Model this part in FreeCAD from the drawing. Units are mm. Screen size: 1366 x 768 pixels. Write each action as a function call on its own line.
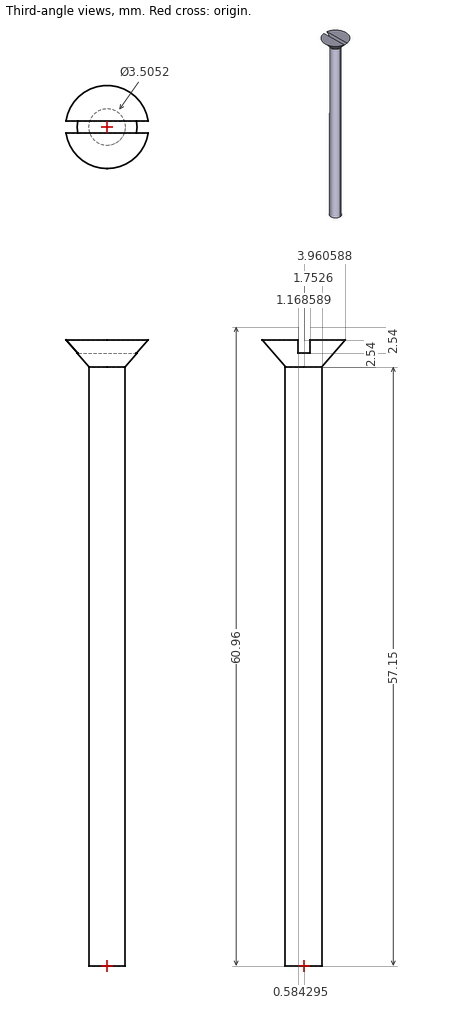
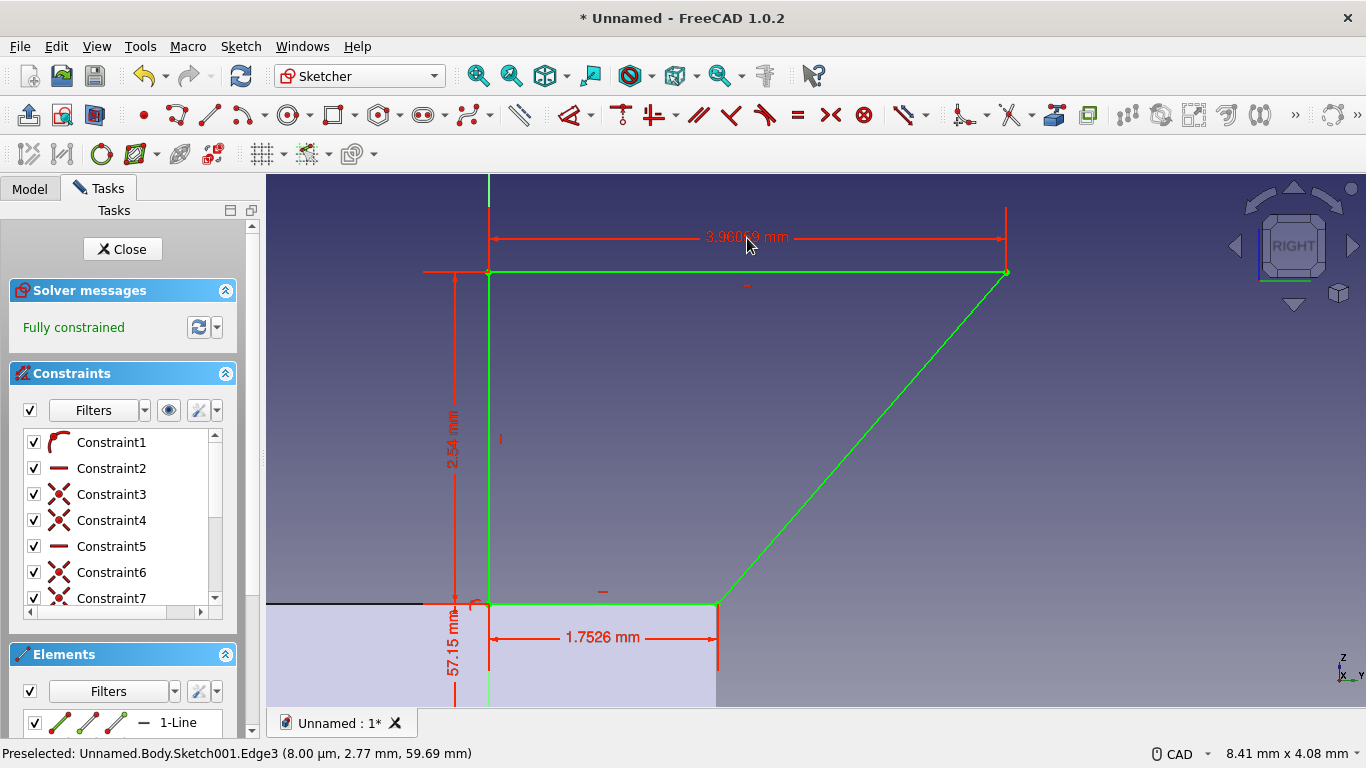
click(123, 249)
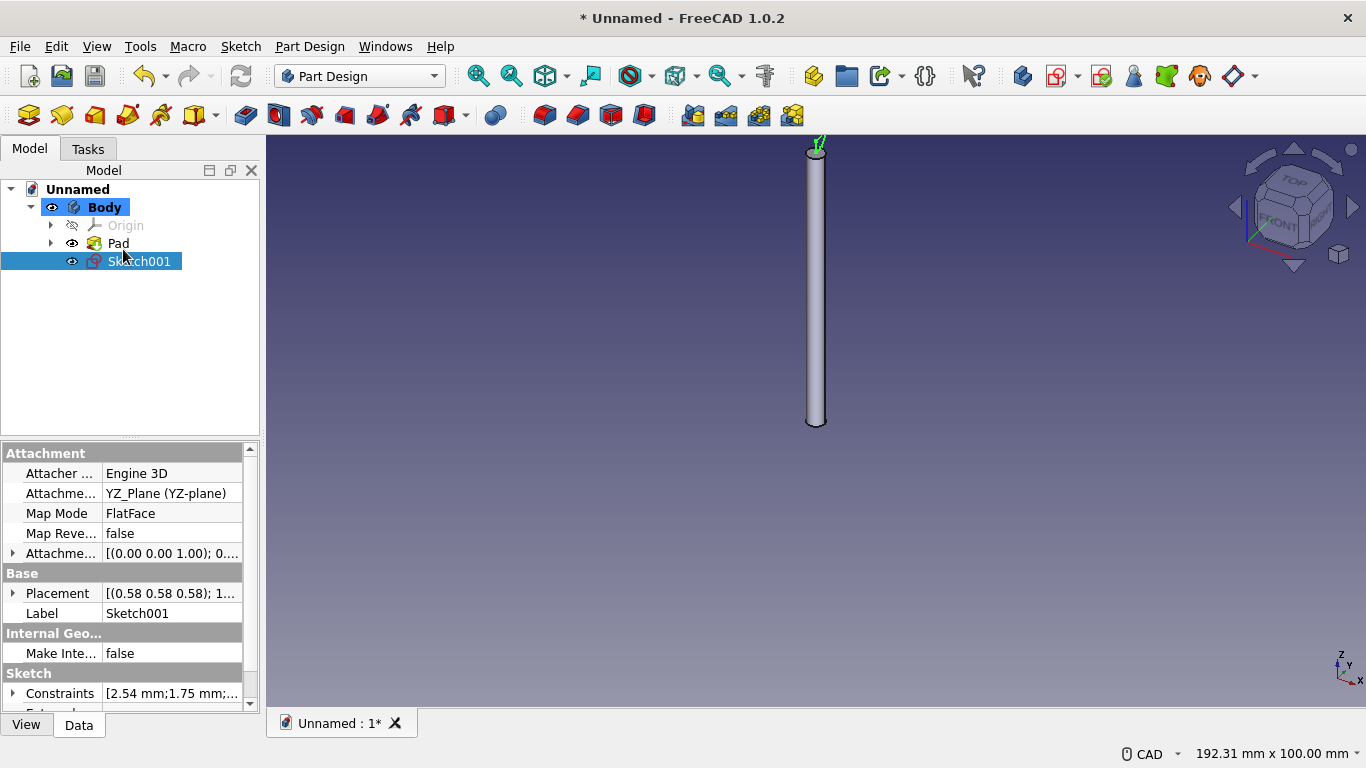
click(62, 116)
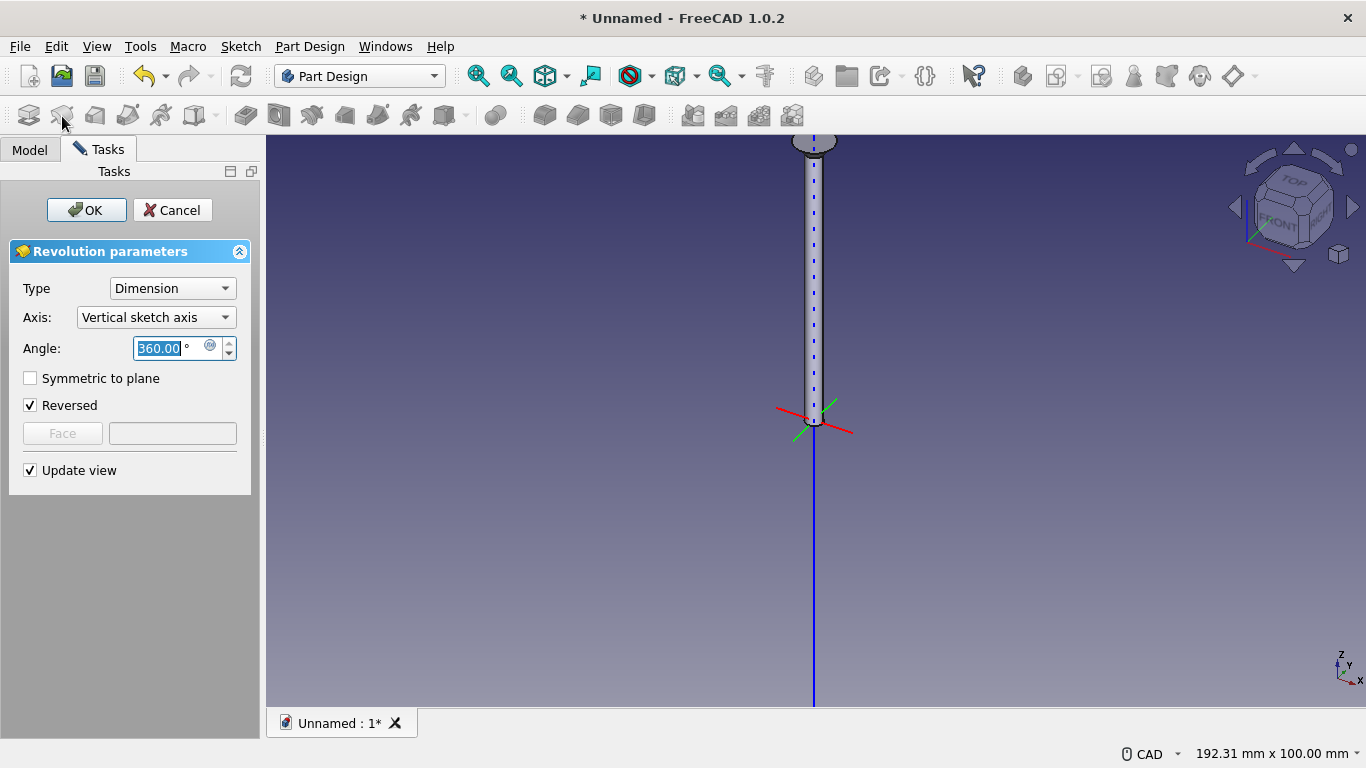
click(87, 210)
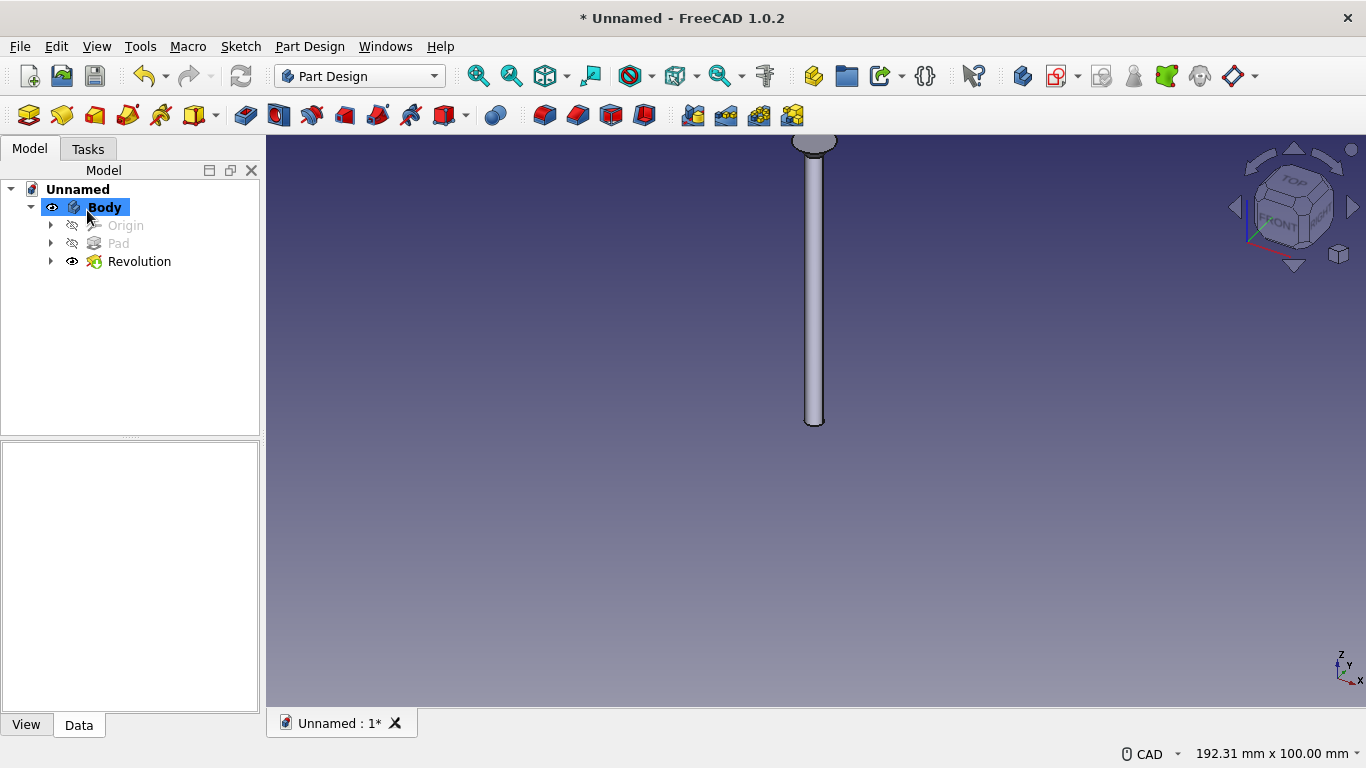
click(479, 76)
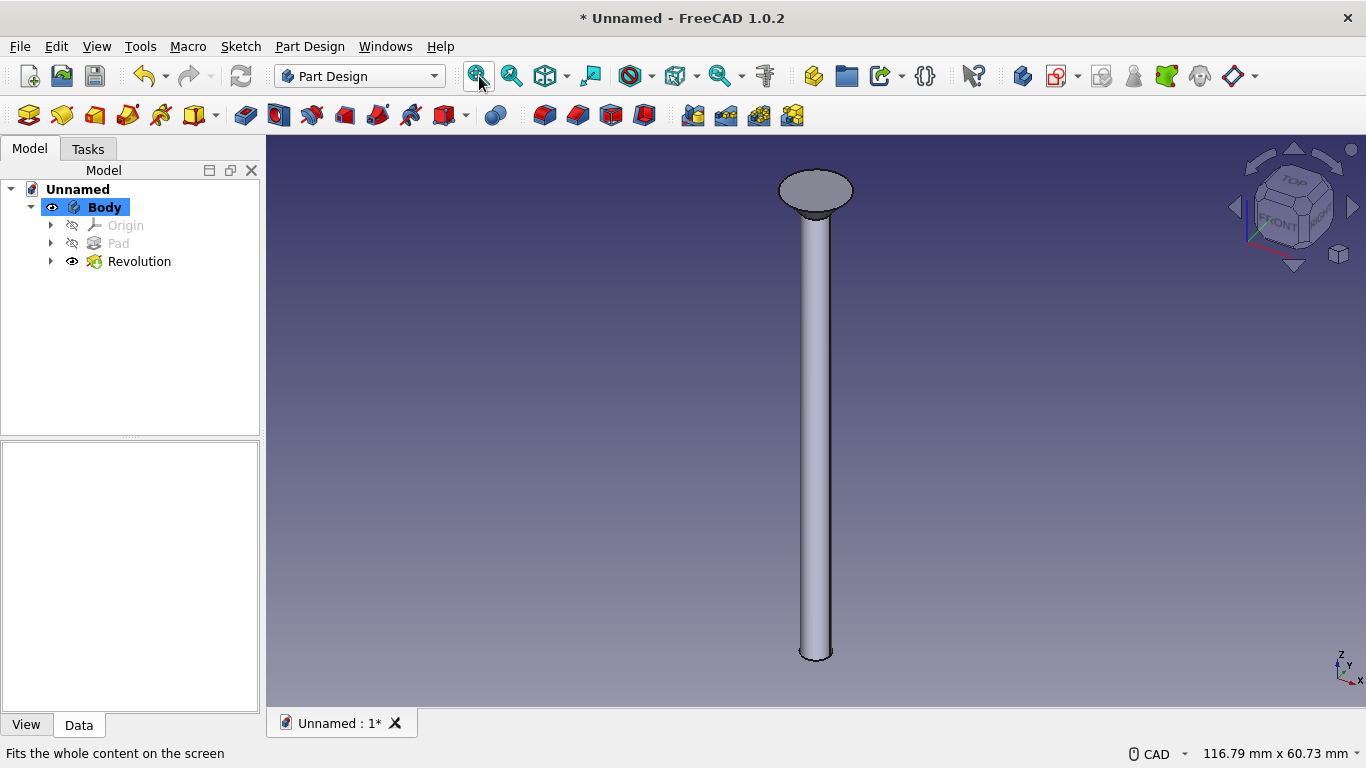
click(1056, 76)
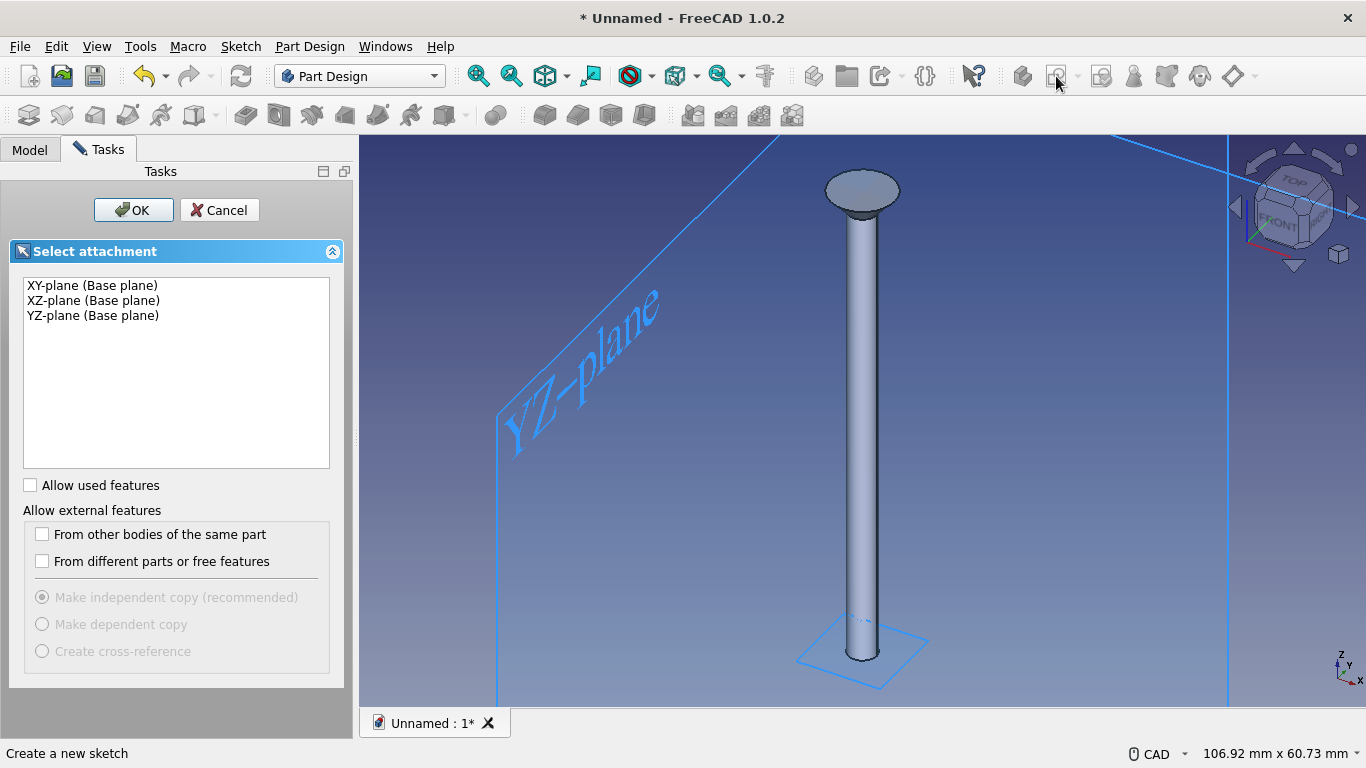
click(84, 316)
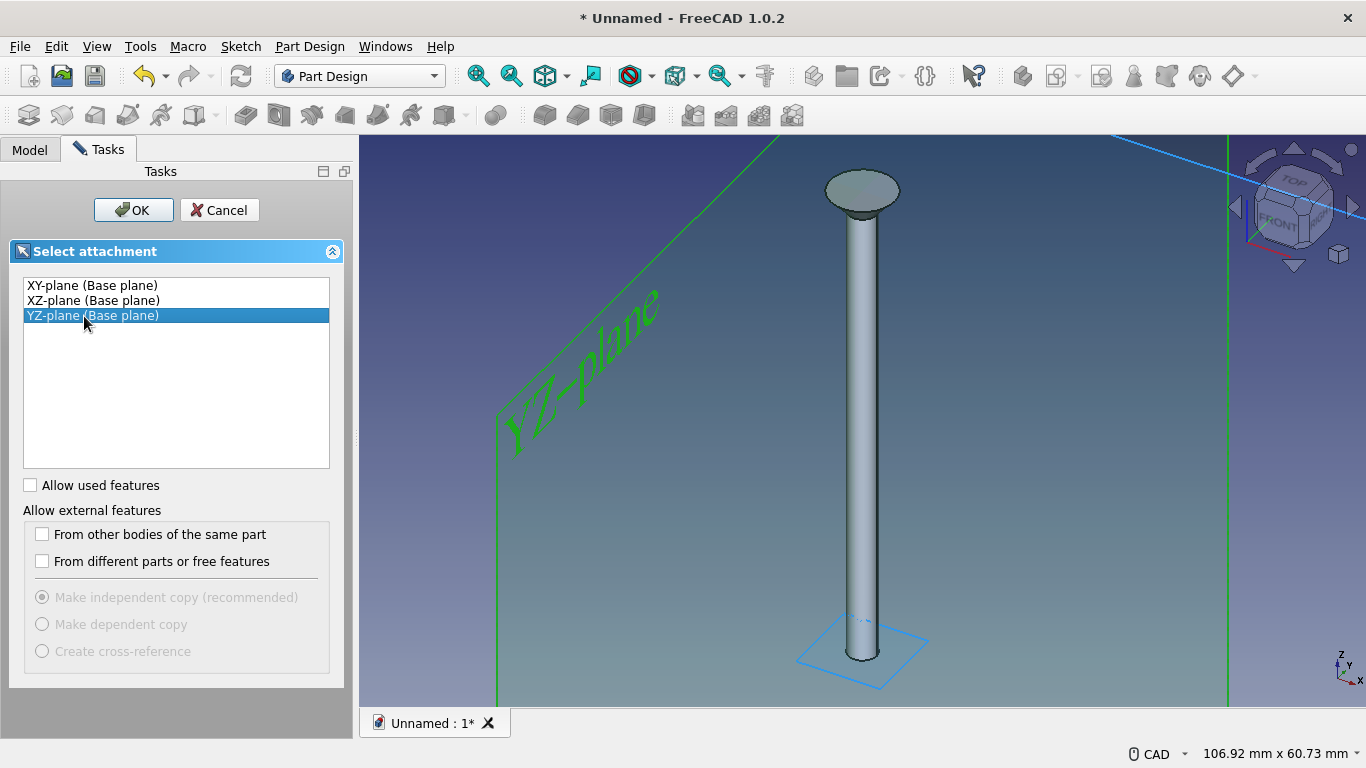
click(134, 210)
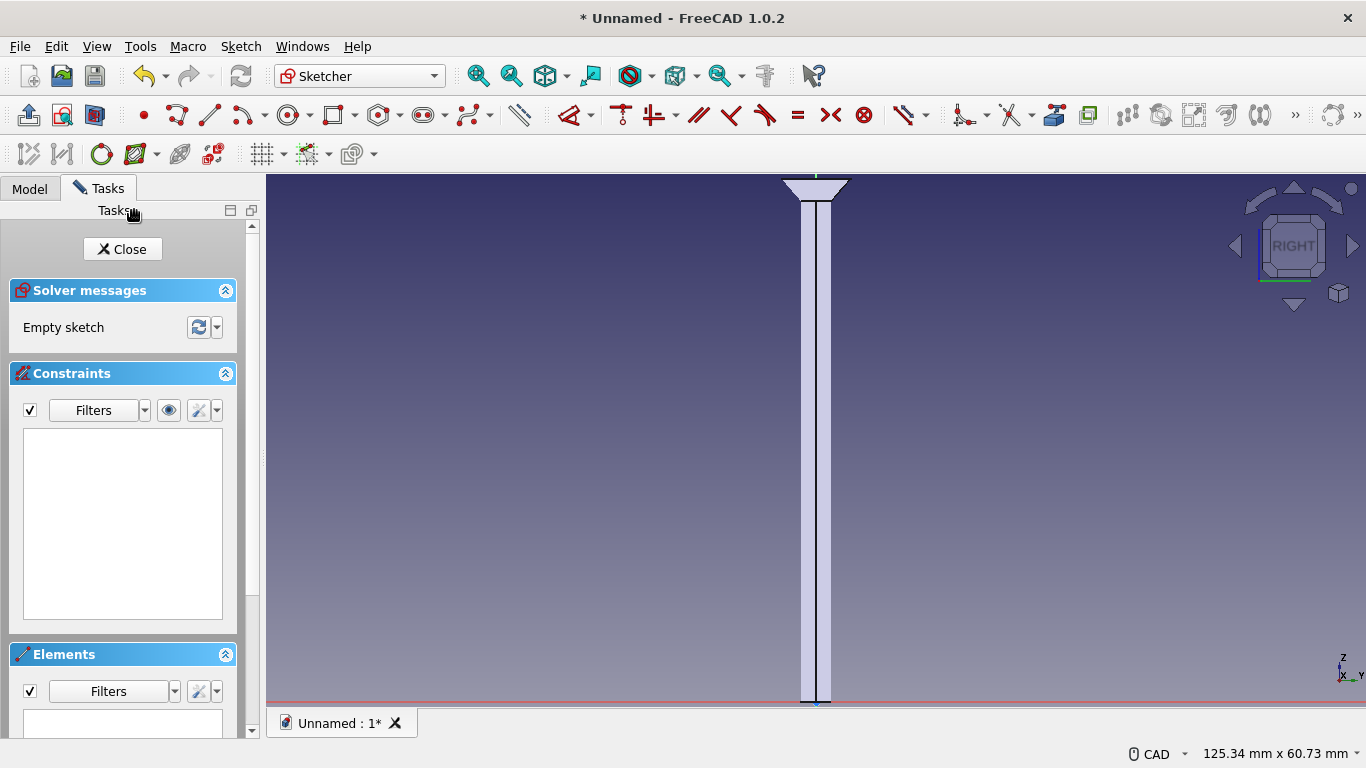
click(95, 116)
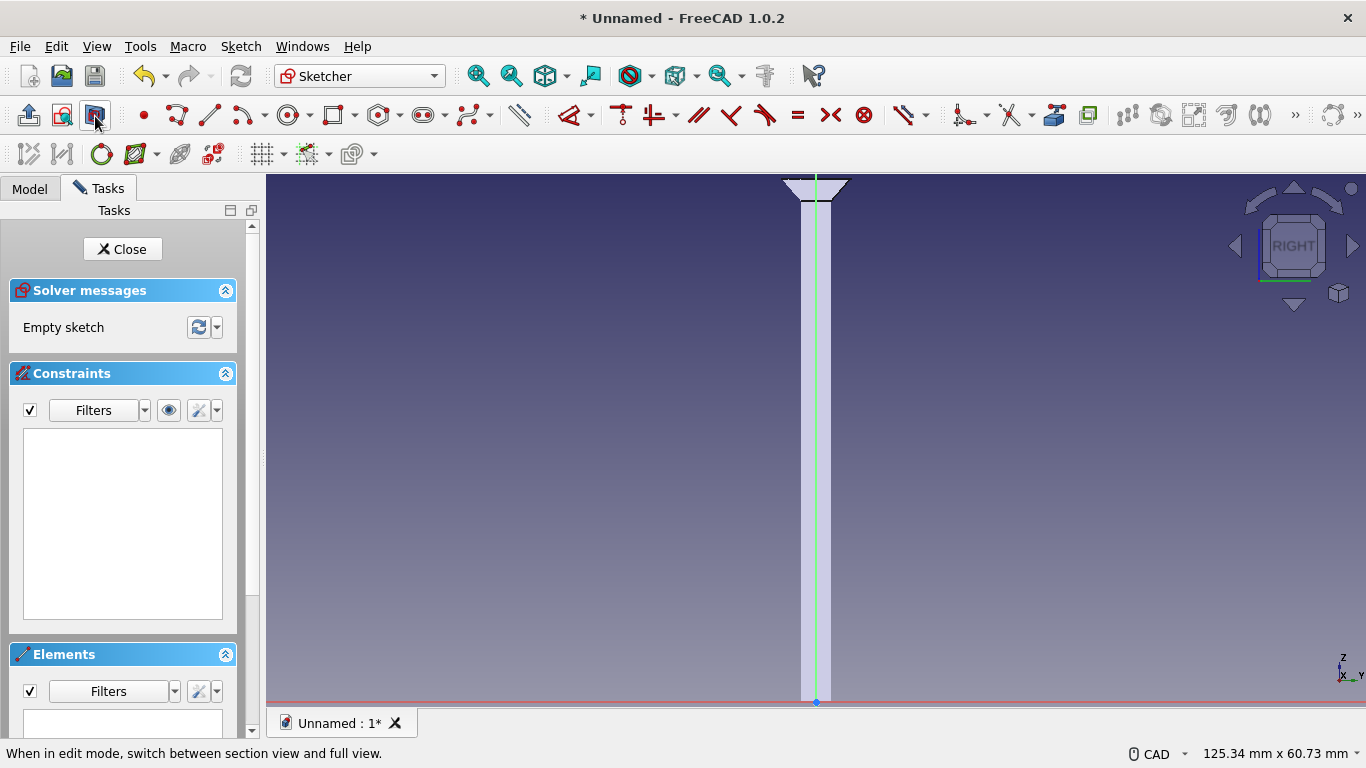
scroll(748, 440, down, 5)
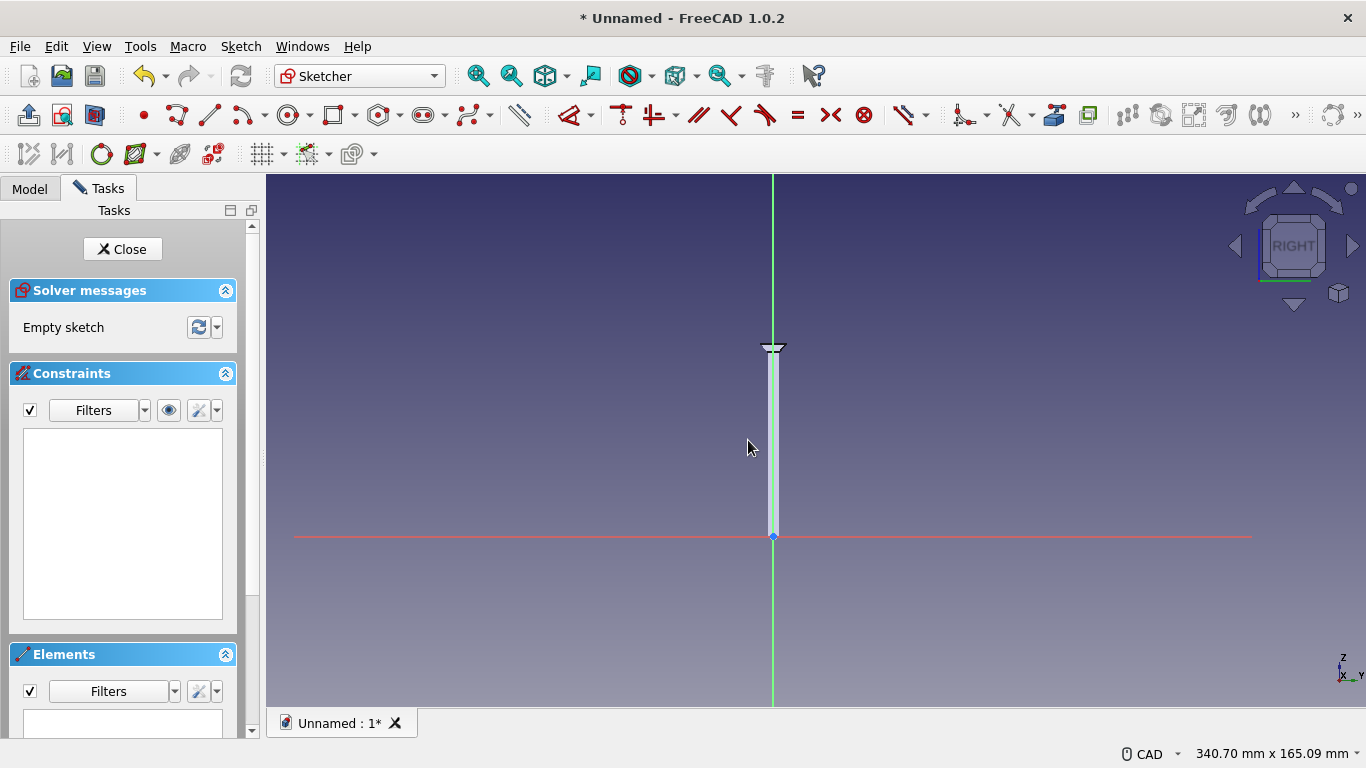
scroll(775, 339, up, 15)